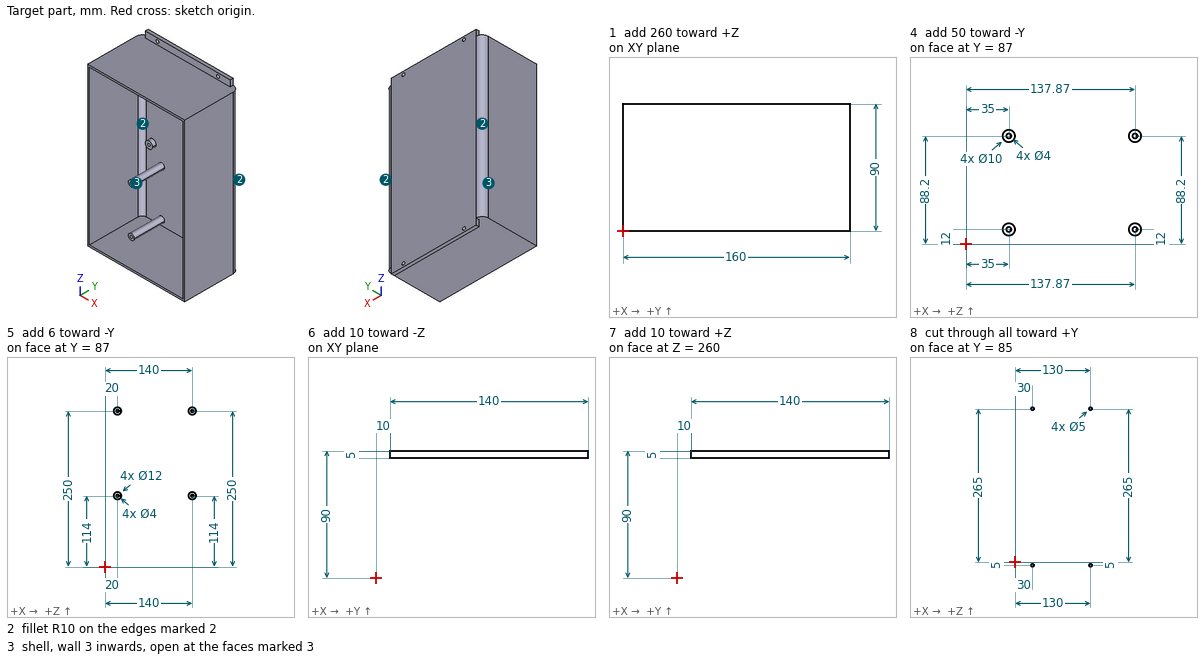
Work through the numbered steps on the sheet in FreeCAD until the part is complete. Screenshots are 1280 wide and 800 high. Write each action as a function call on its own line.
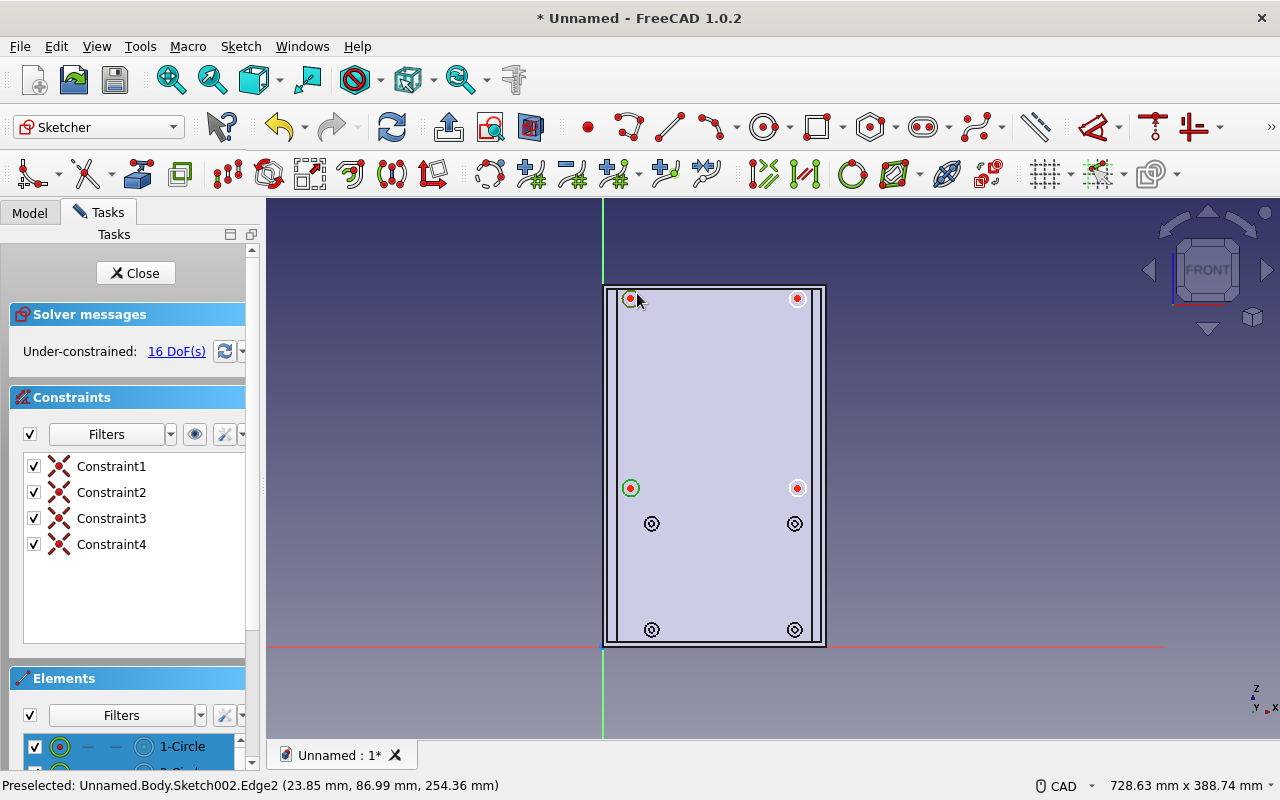
scroll(804, 482, up, 5)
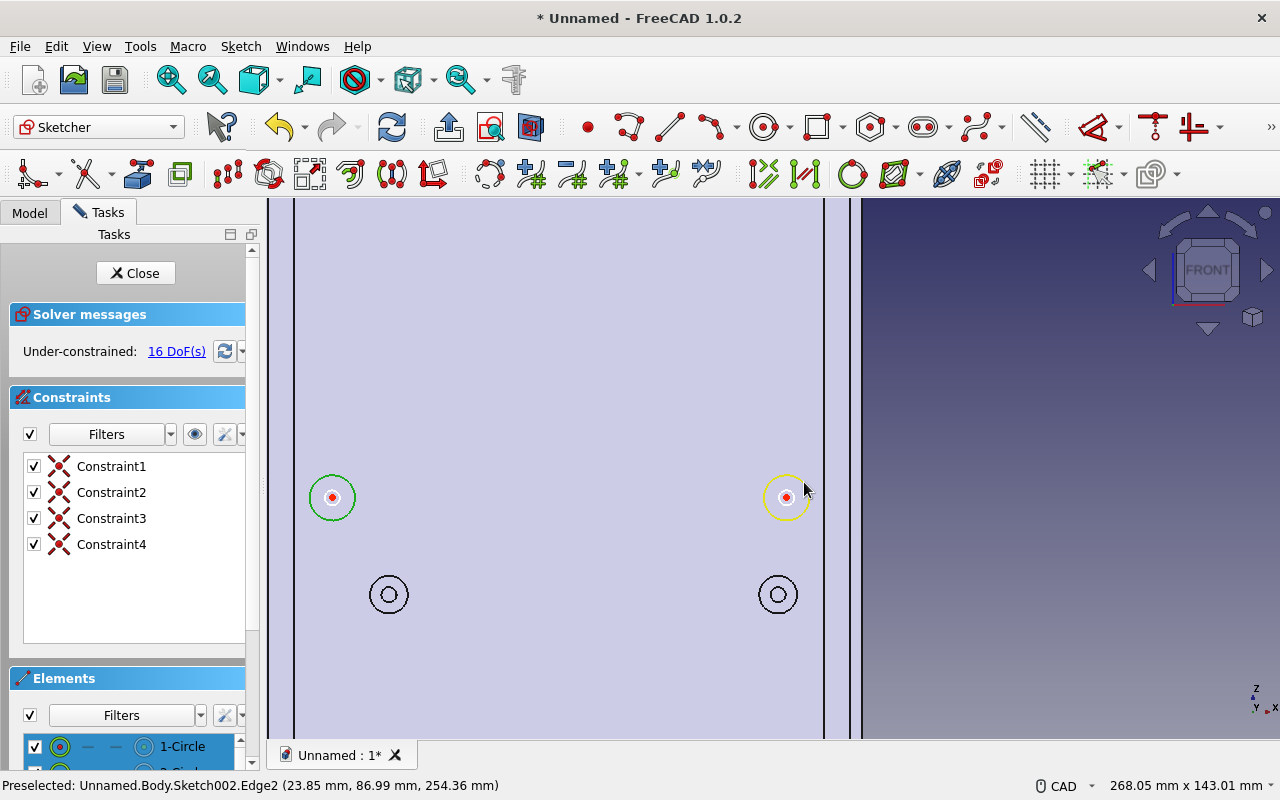
click(803, 482)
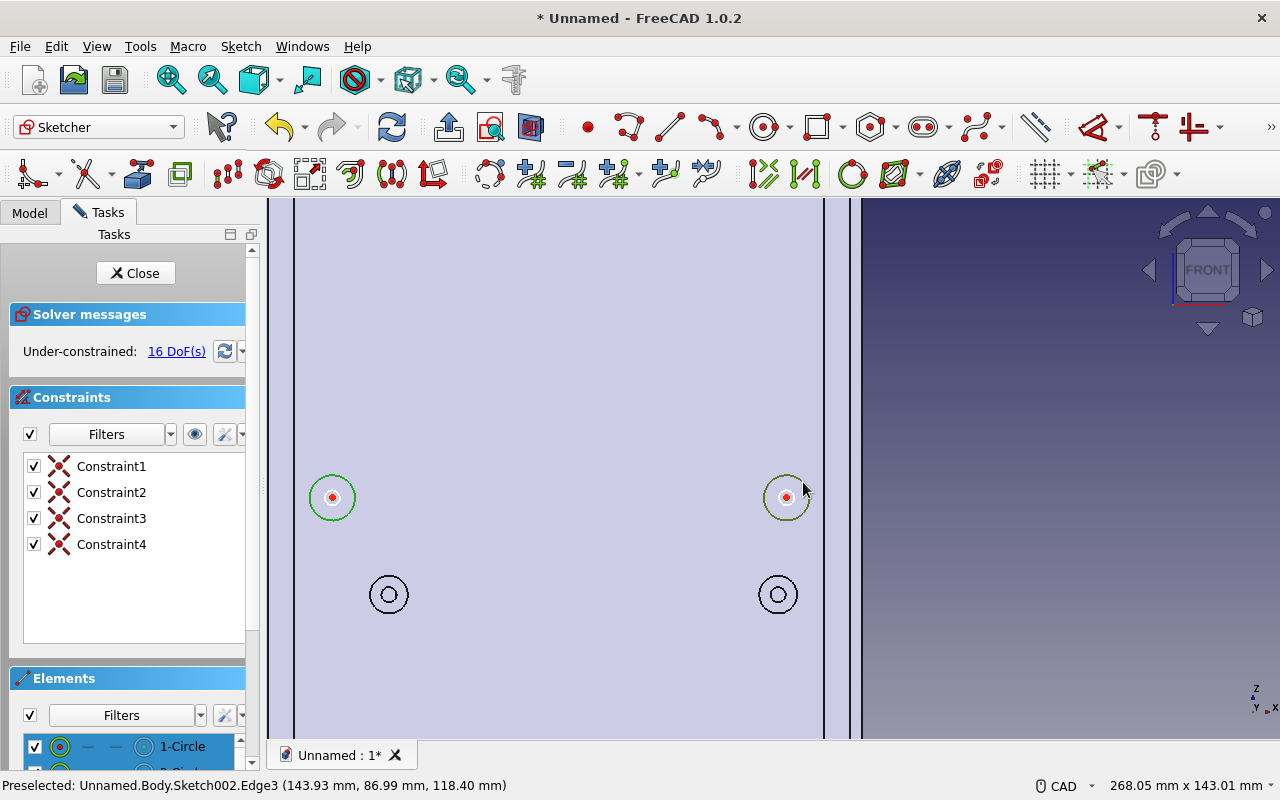
scroll(804, 483, down, 5)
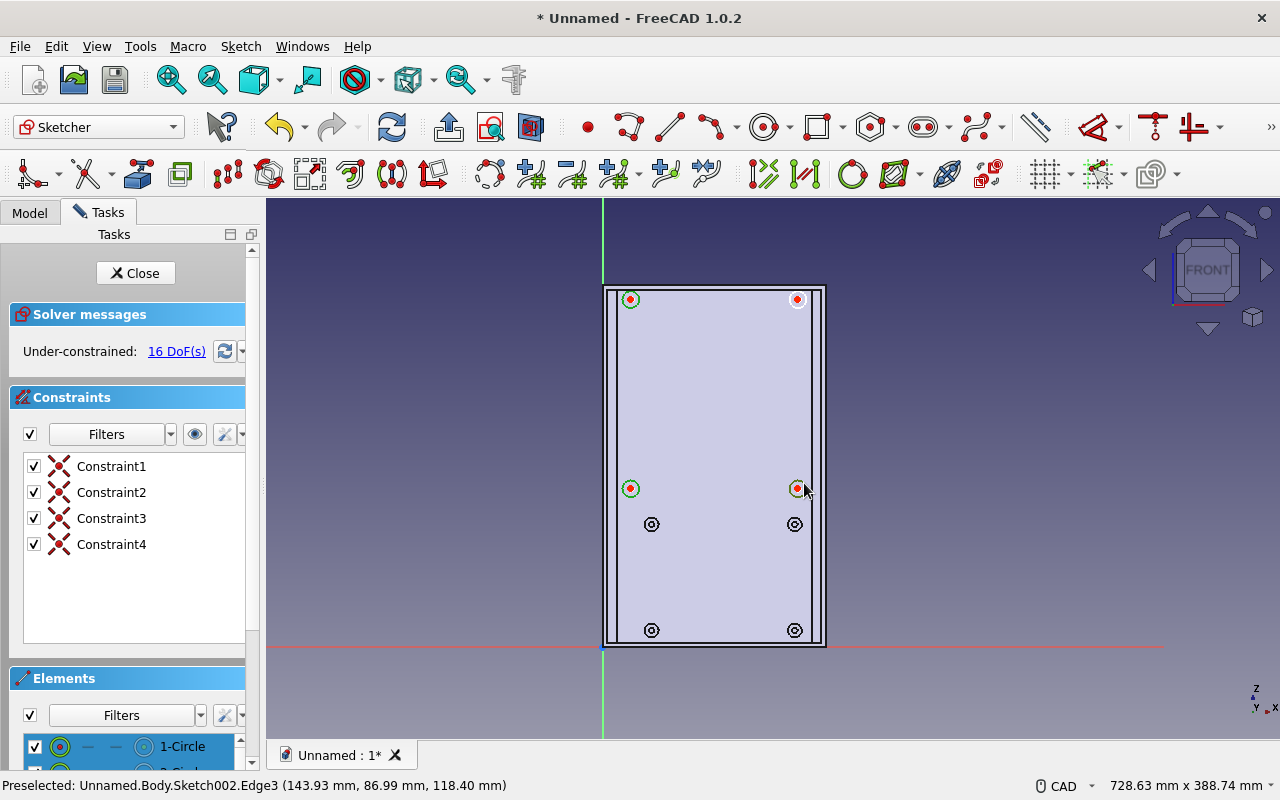
scroll(804, 294, up, 5)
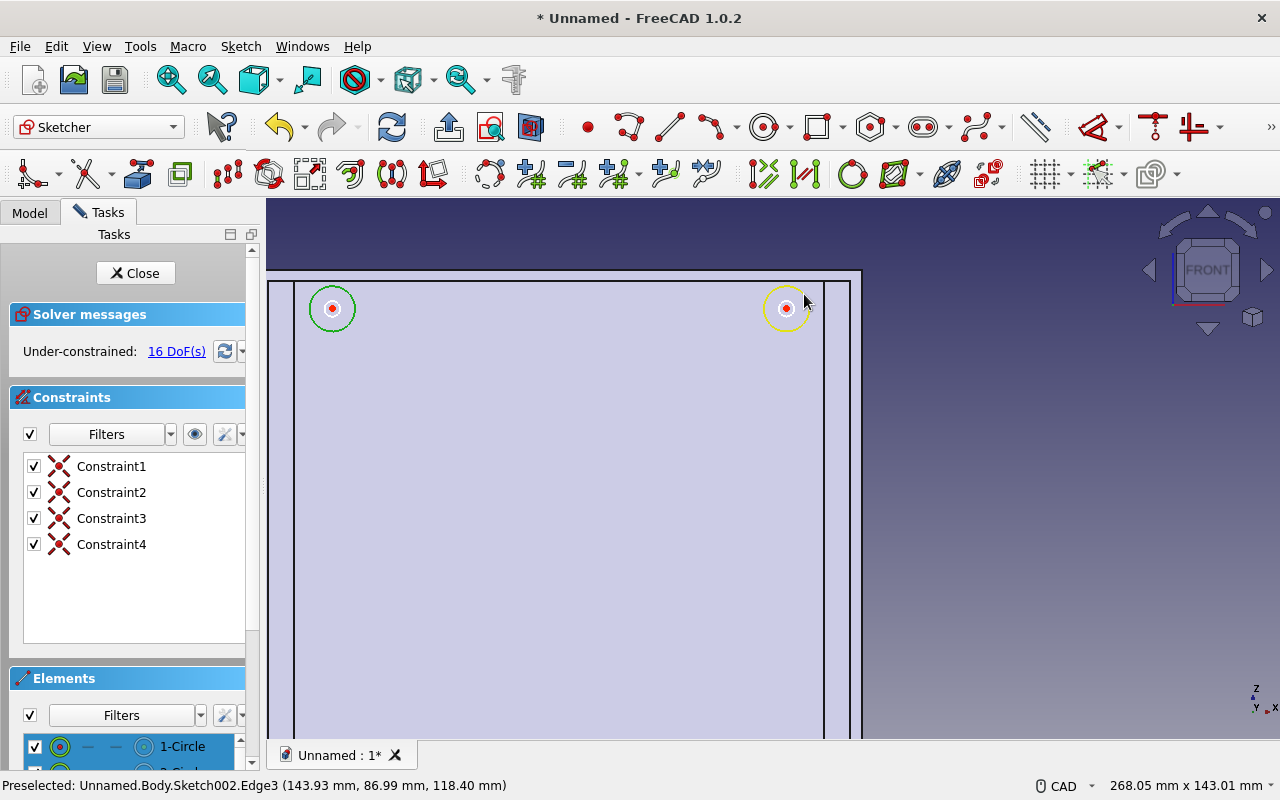
click(803, 293)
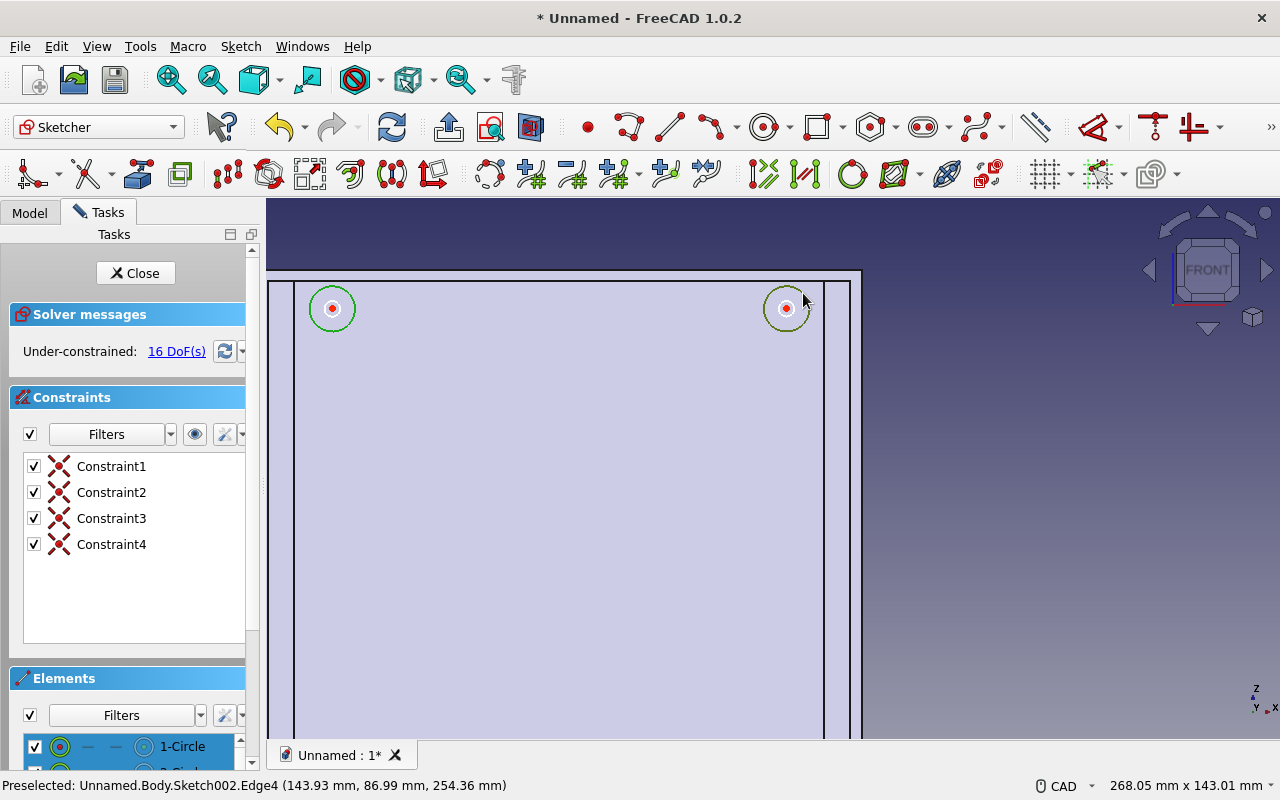
key(e)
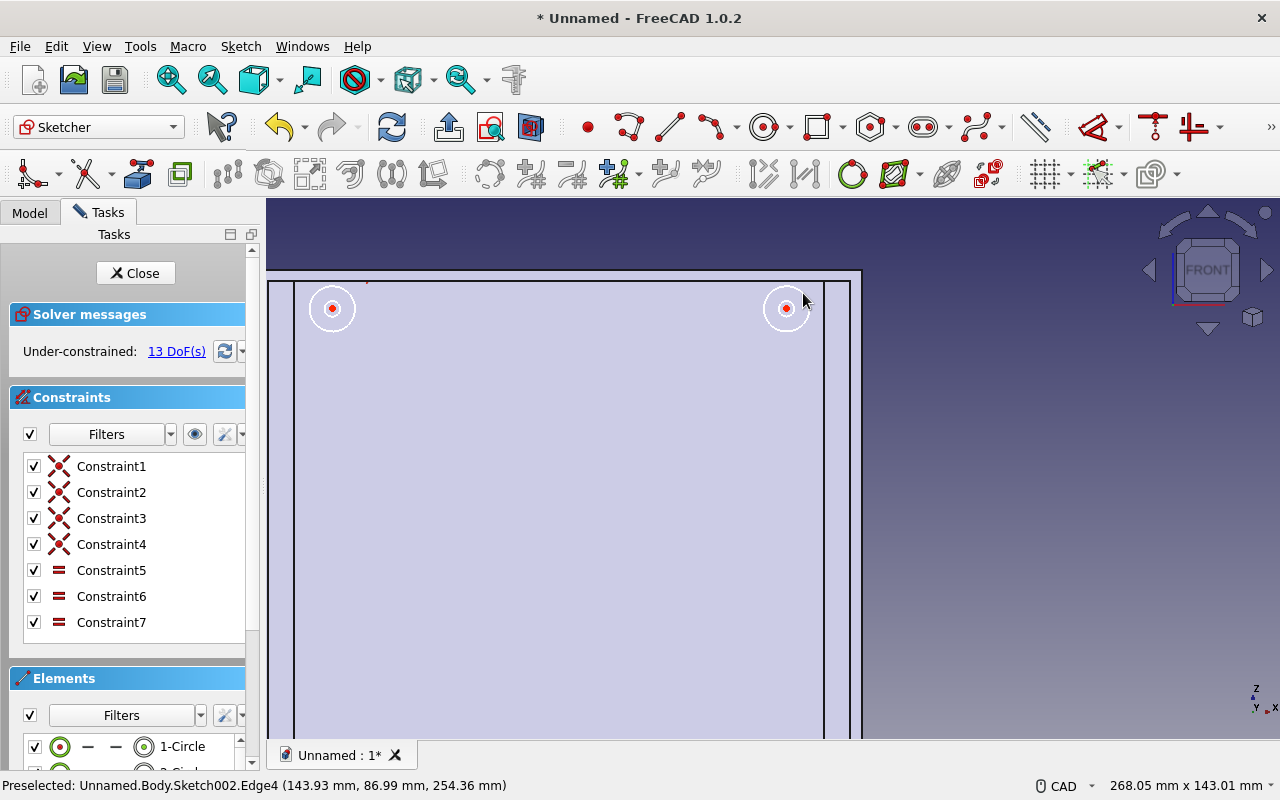
scroll(804, 293, down, 5)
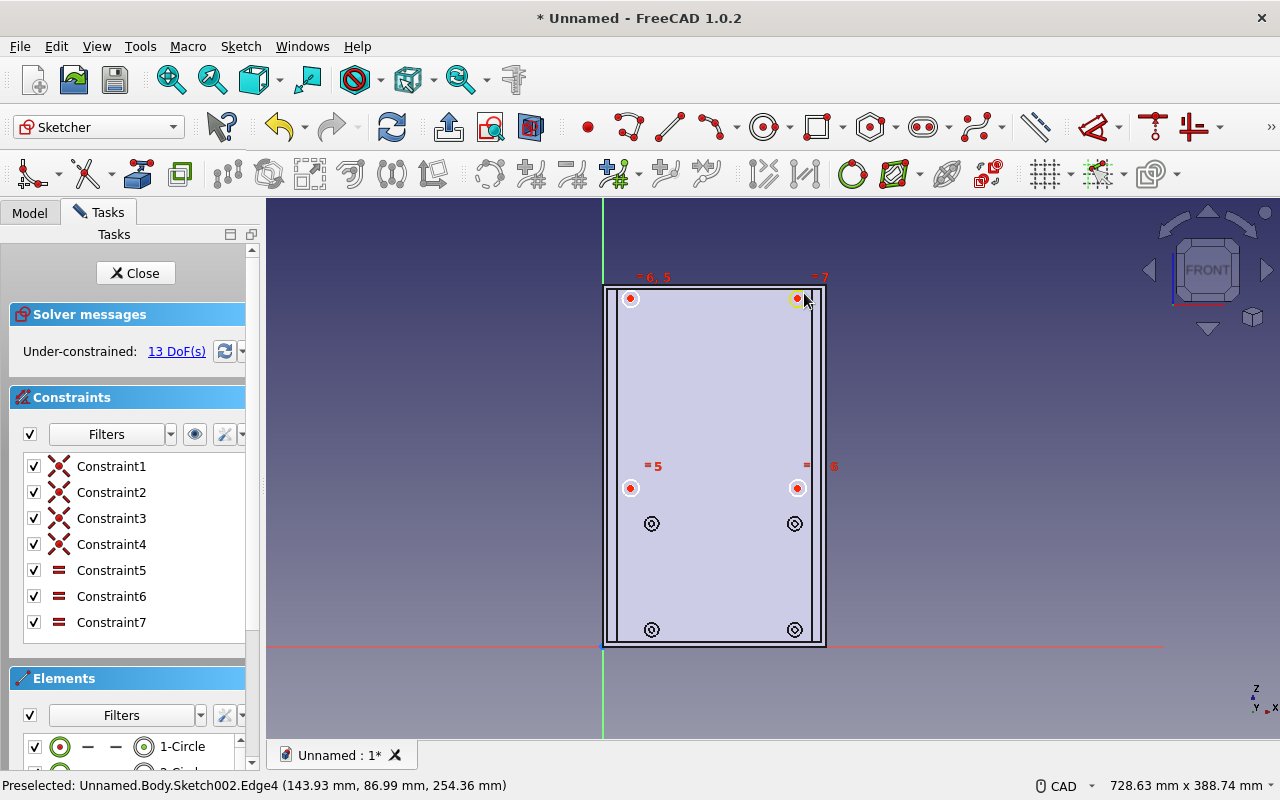
scroll(629, 486, up, 9)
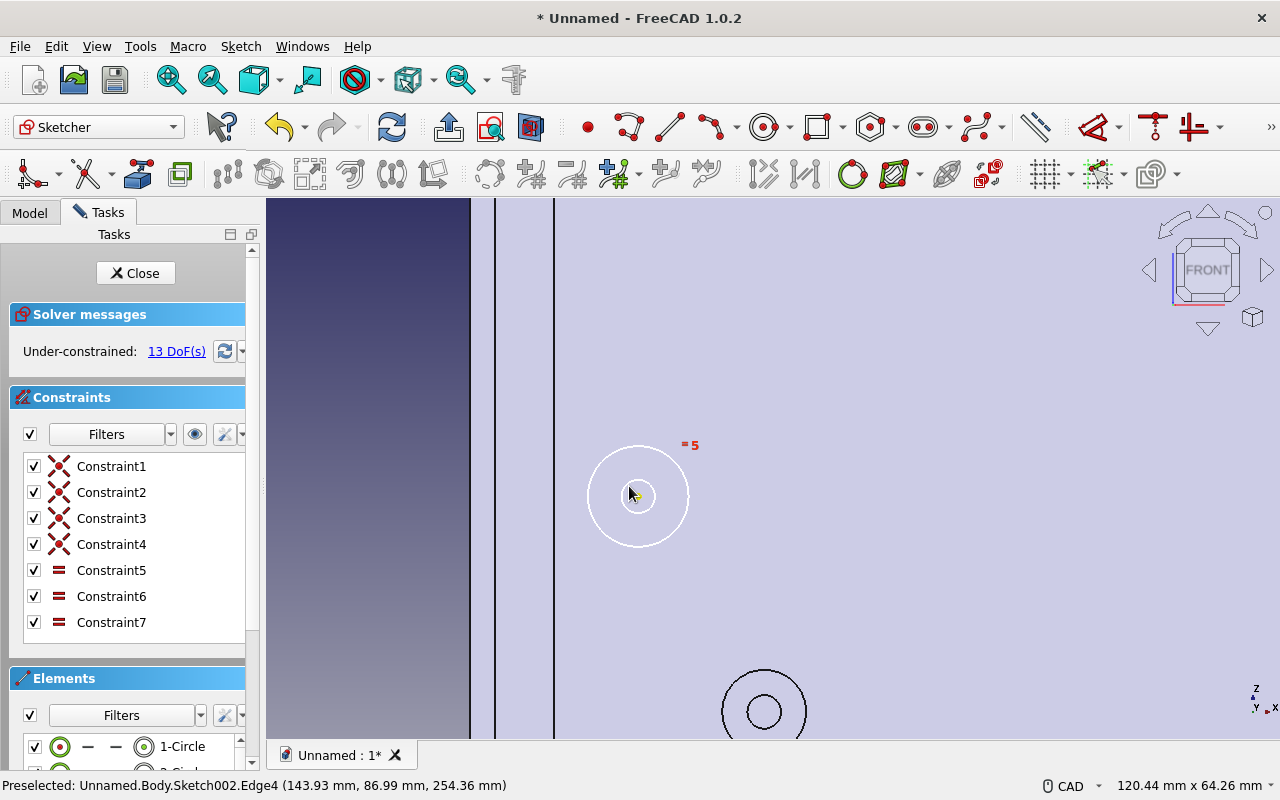
click(626, 485)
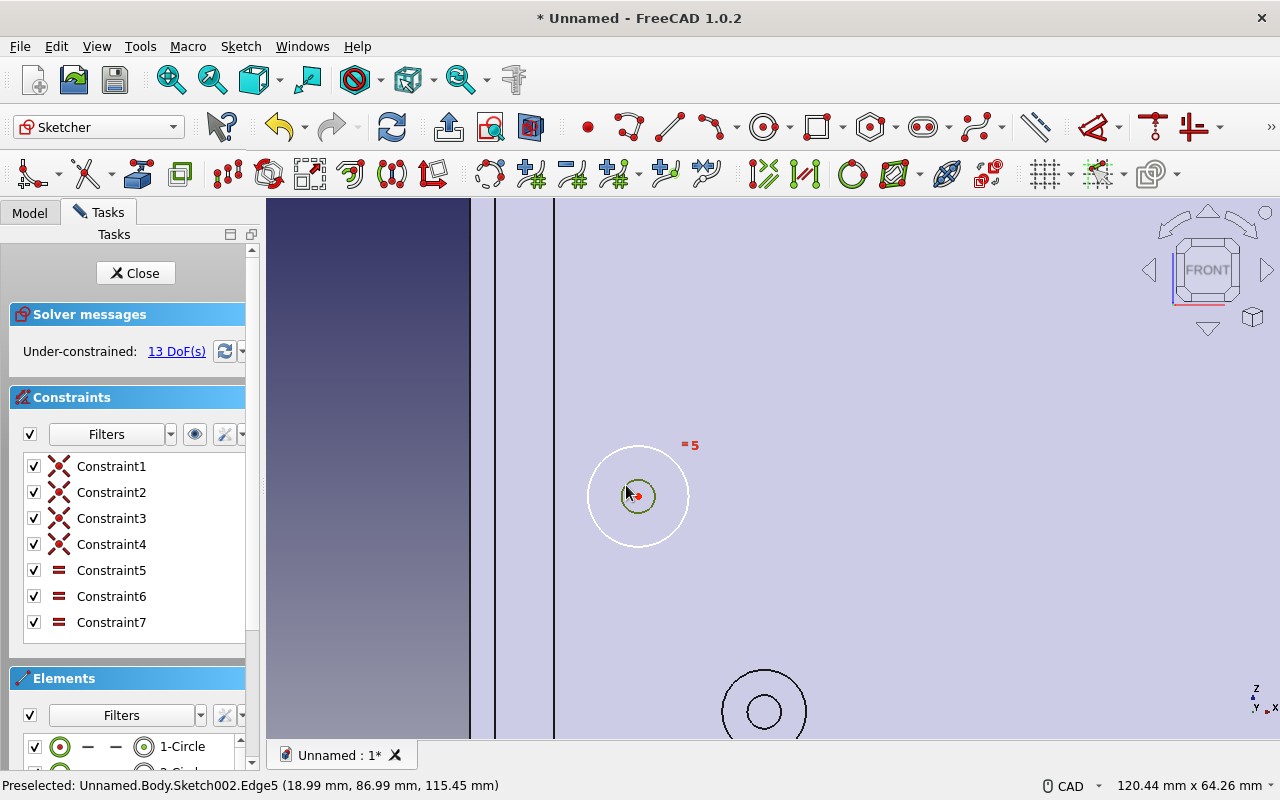
scroll(629, 487, down, 9)